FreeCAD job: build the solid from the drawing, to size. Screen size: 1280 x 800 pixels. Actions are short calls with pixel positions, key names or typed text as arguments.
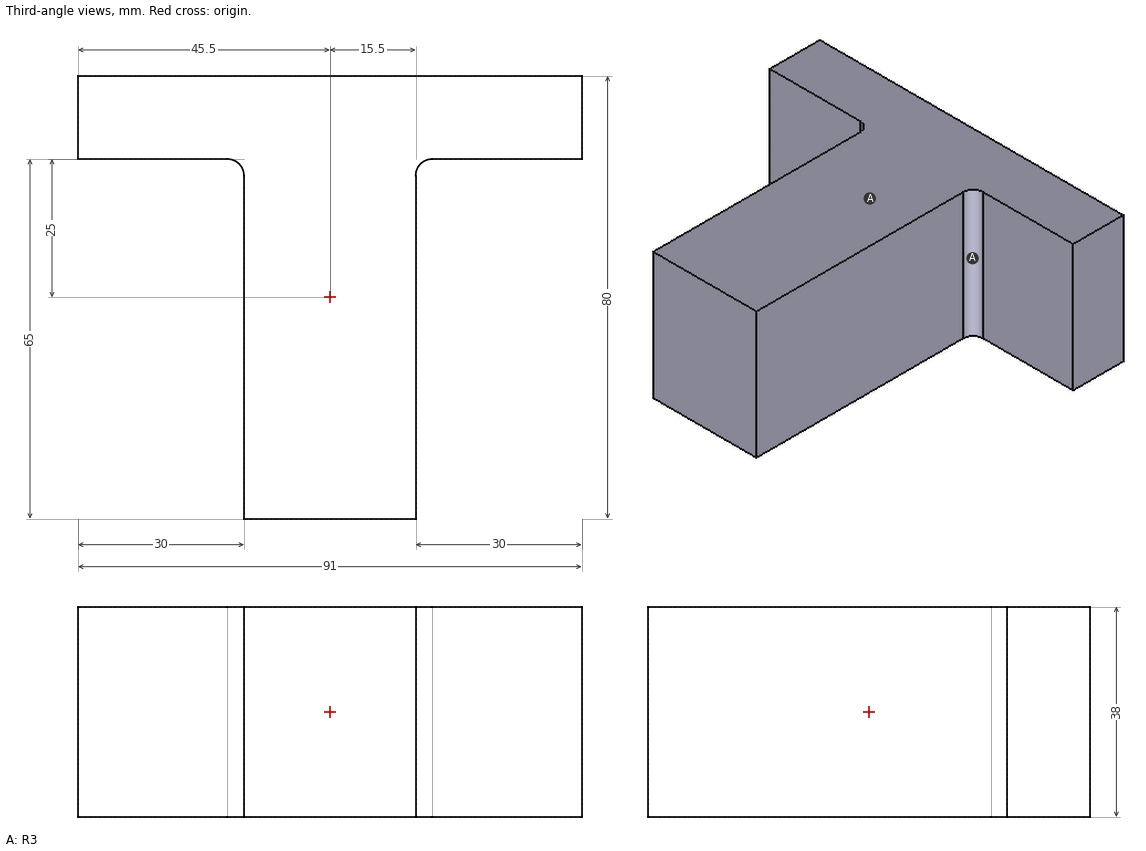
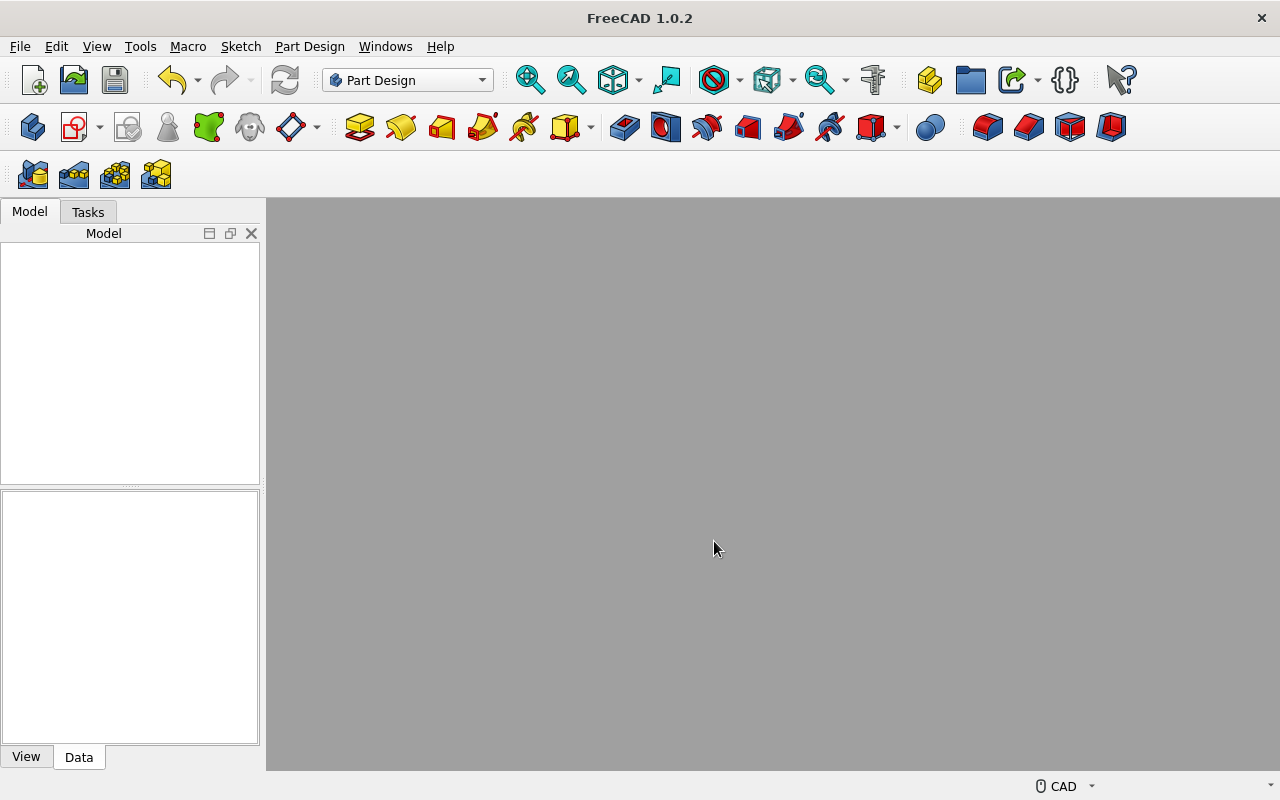
click(33, 80)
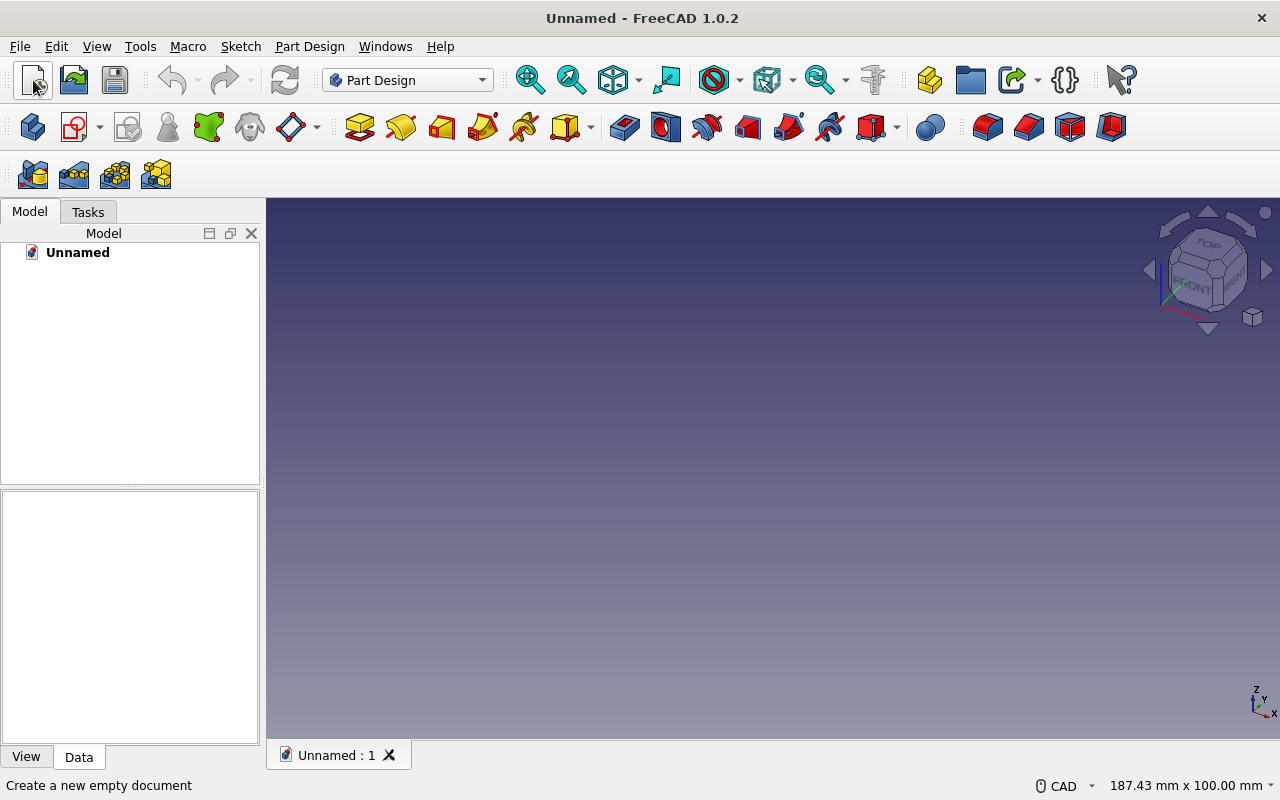
click(74, 128)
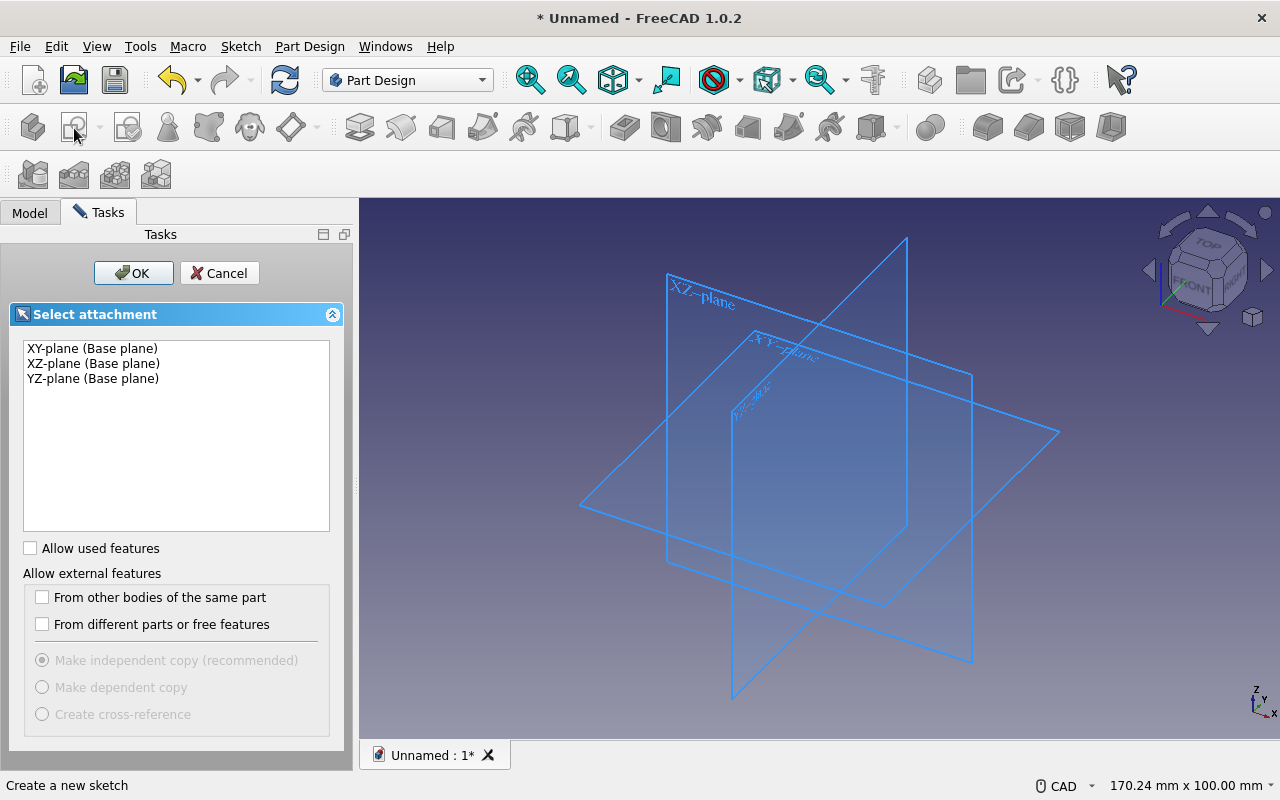
click(84, 348)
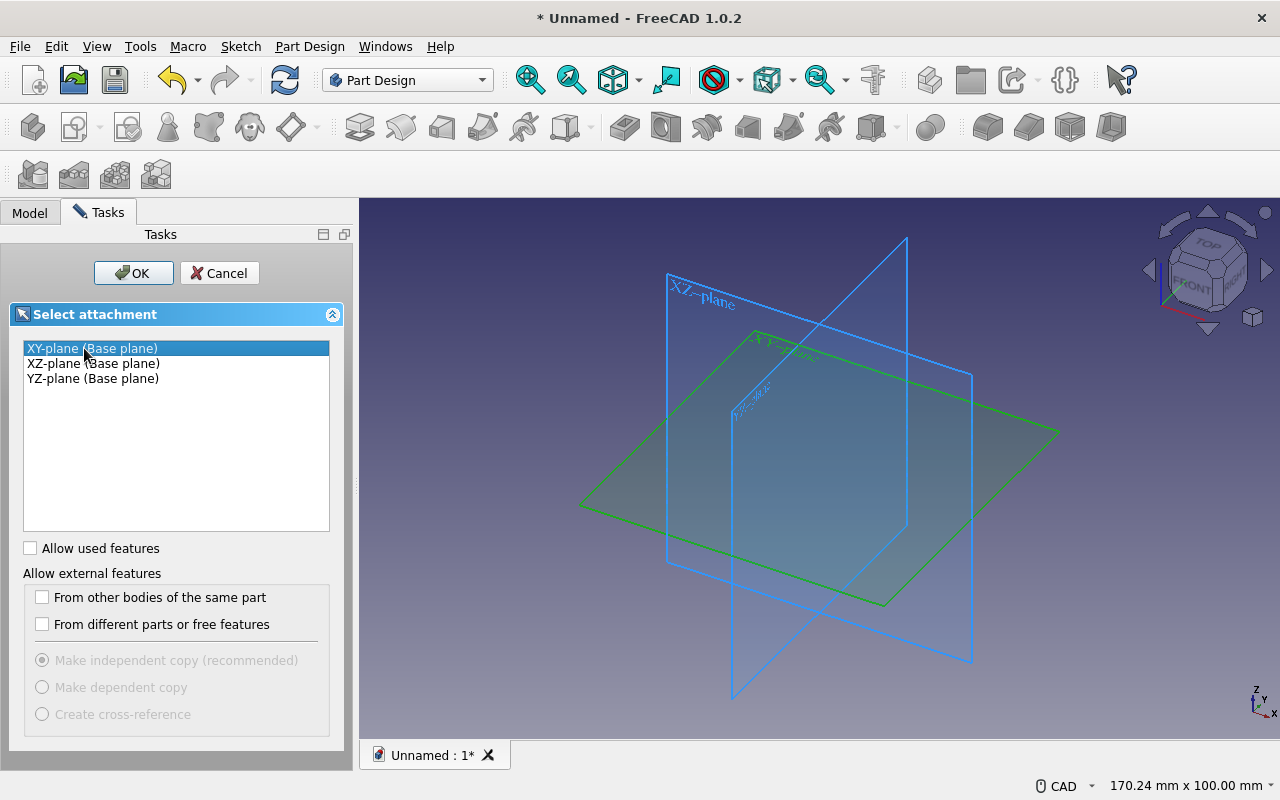
click(134, 273)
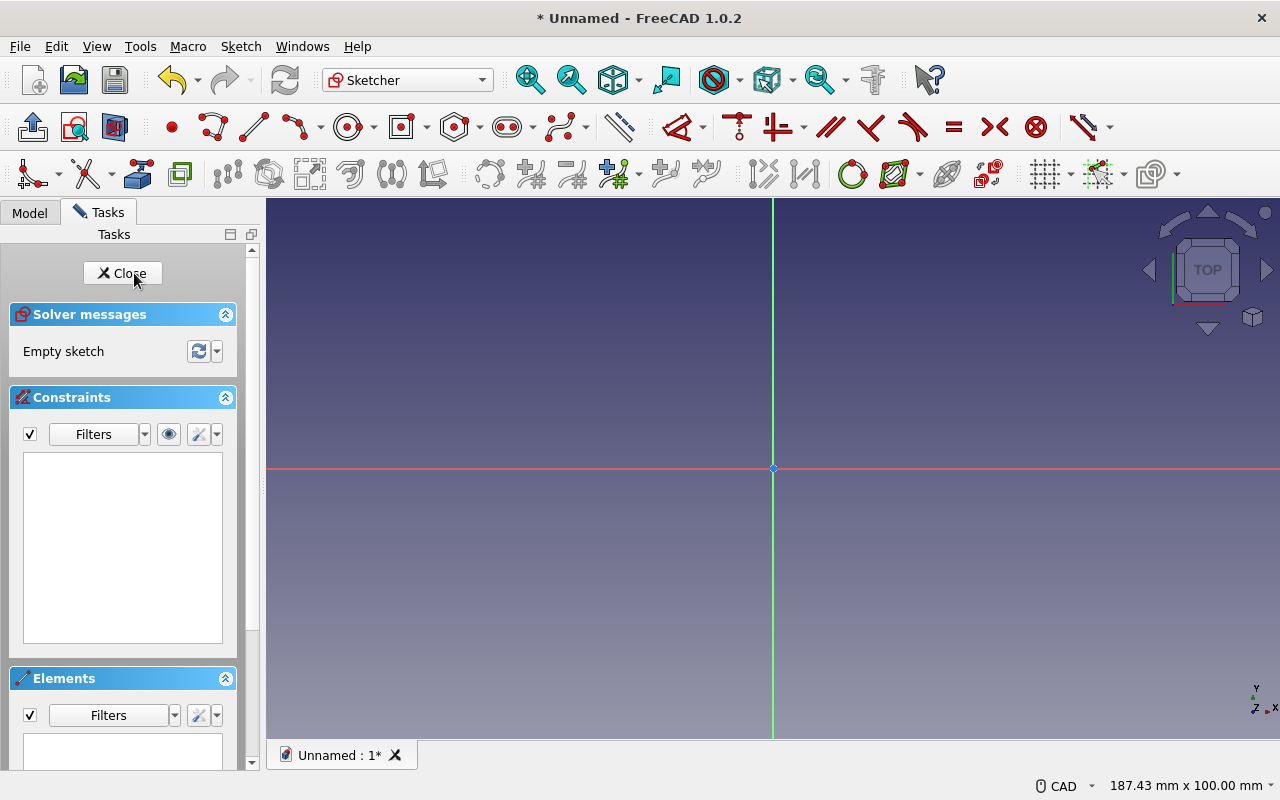
click(400, 128)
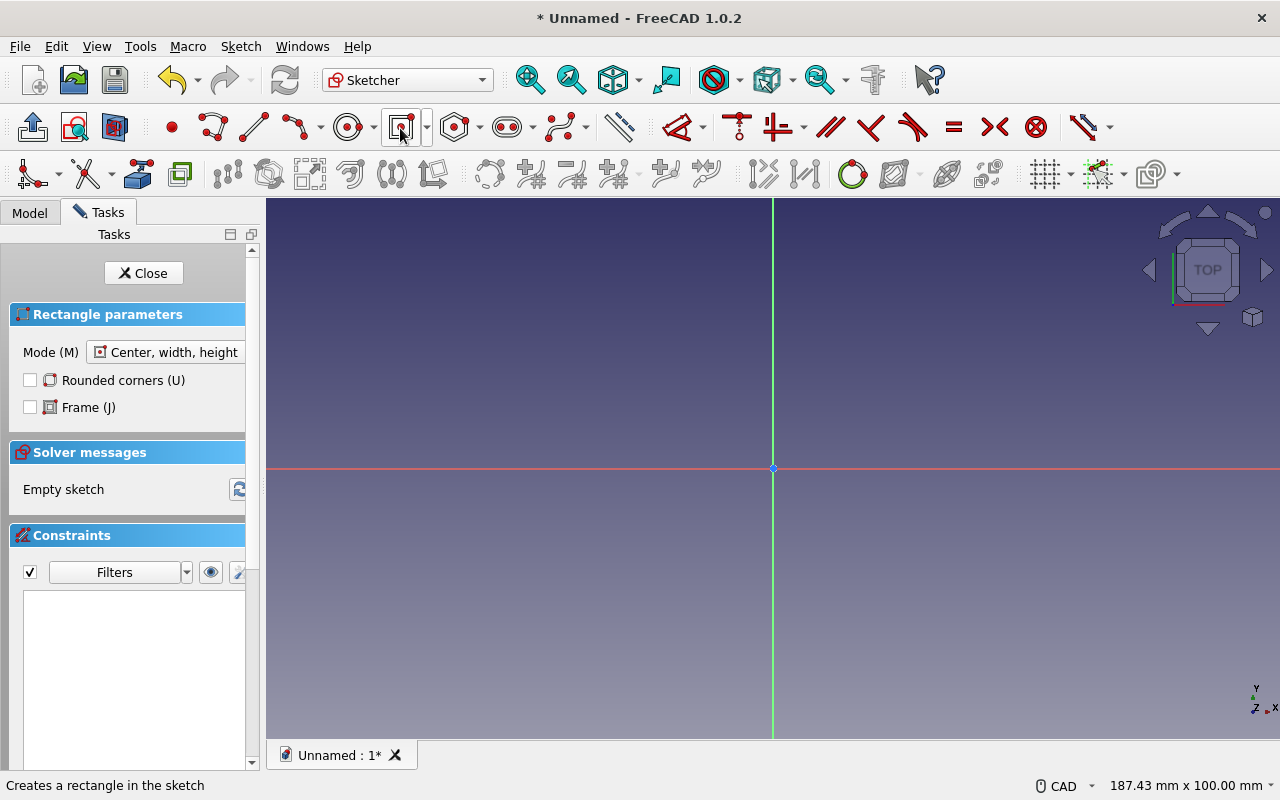
click(773, 468)
move(1019, 252)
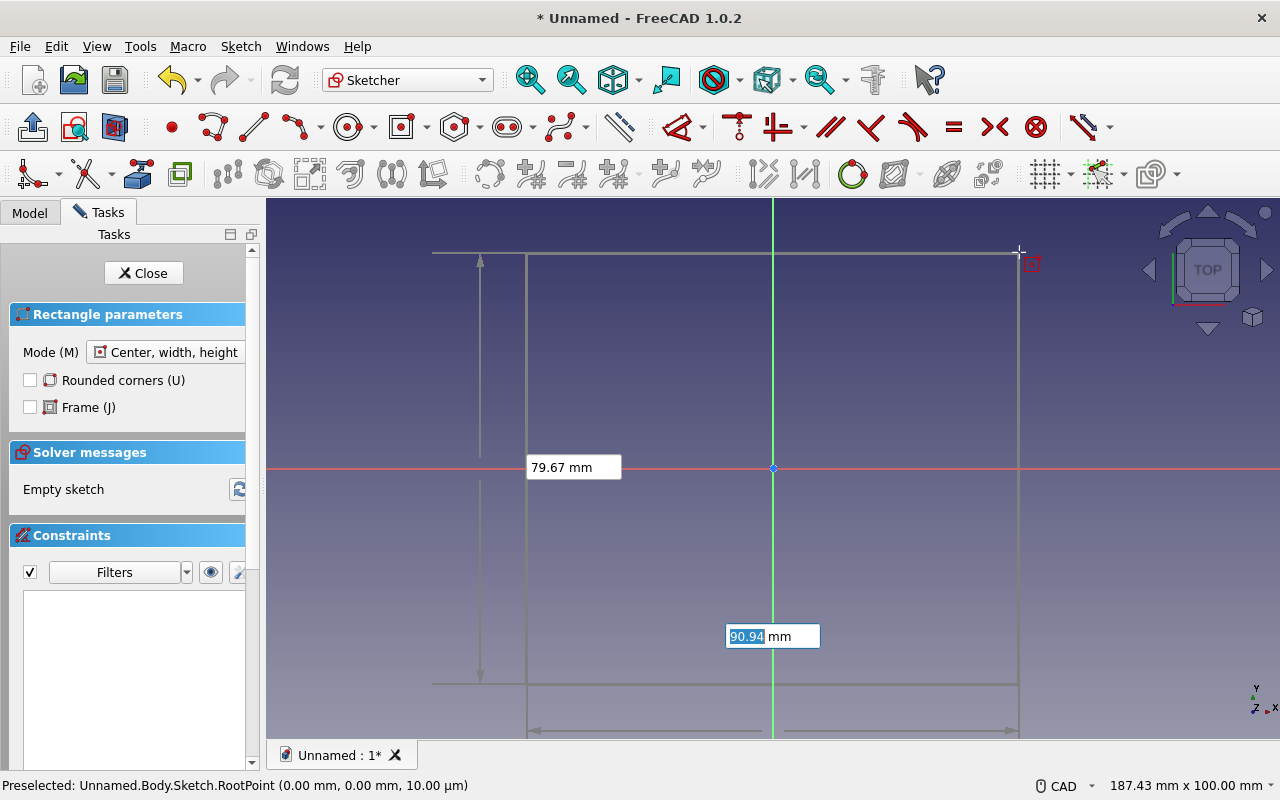
text(91)
key(Tab)
text(80)
key(Return)
key(Escape)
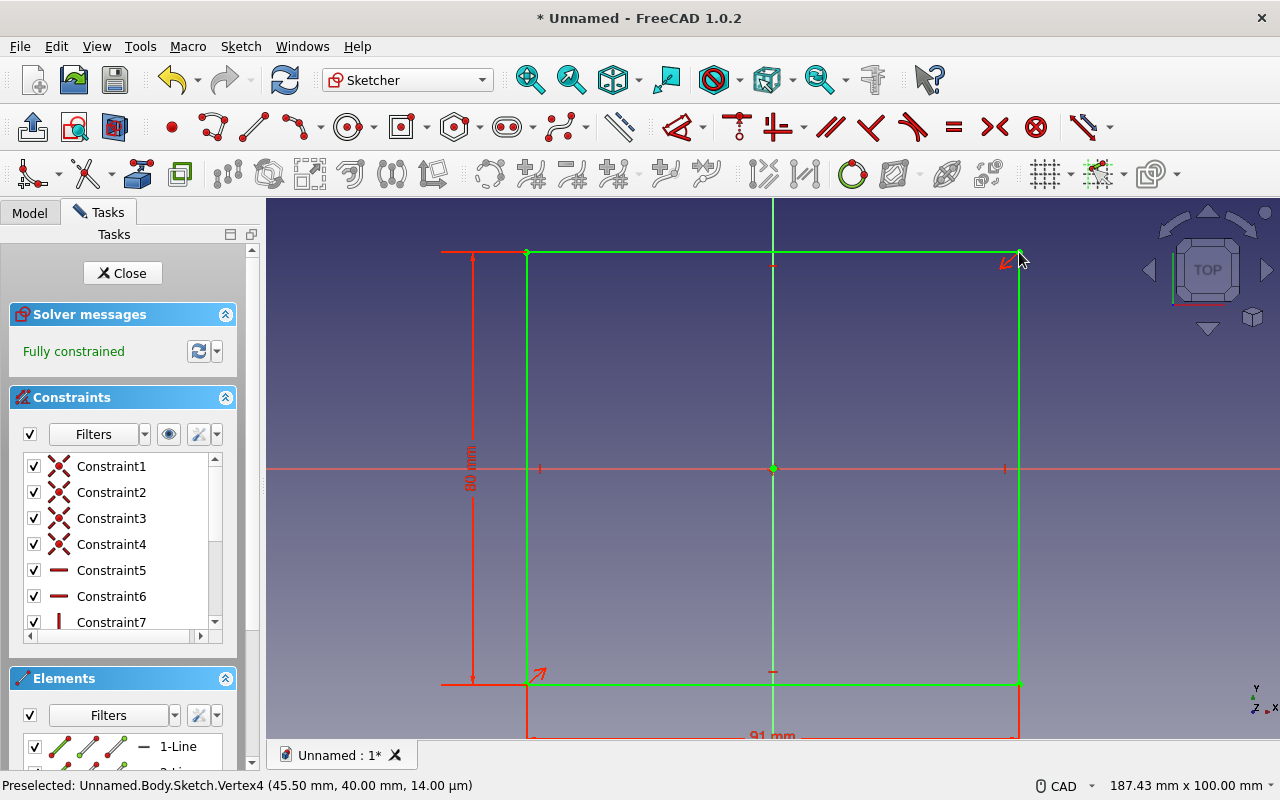
click(123, 273)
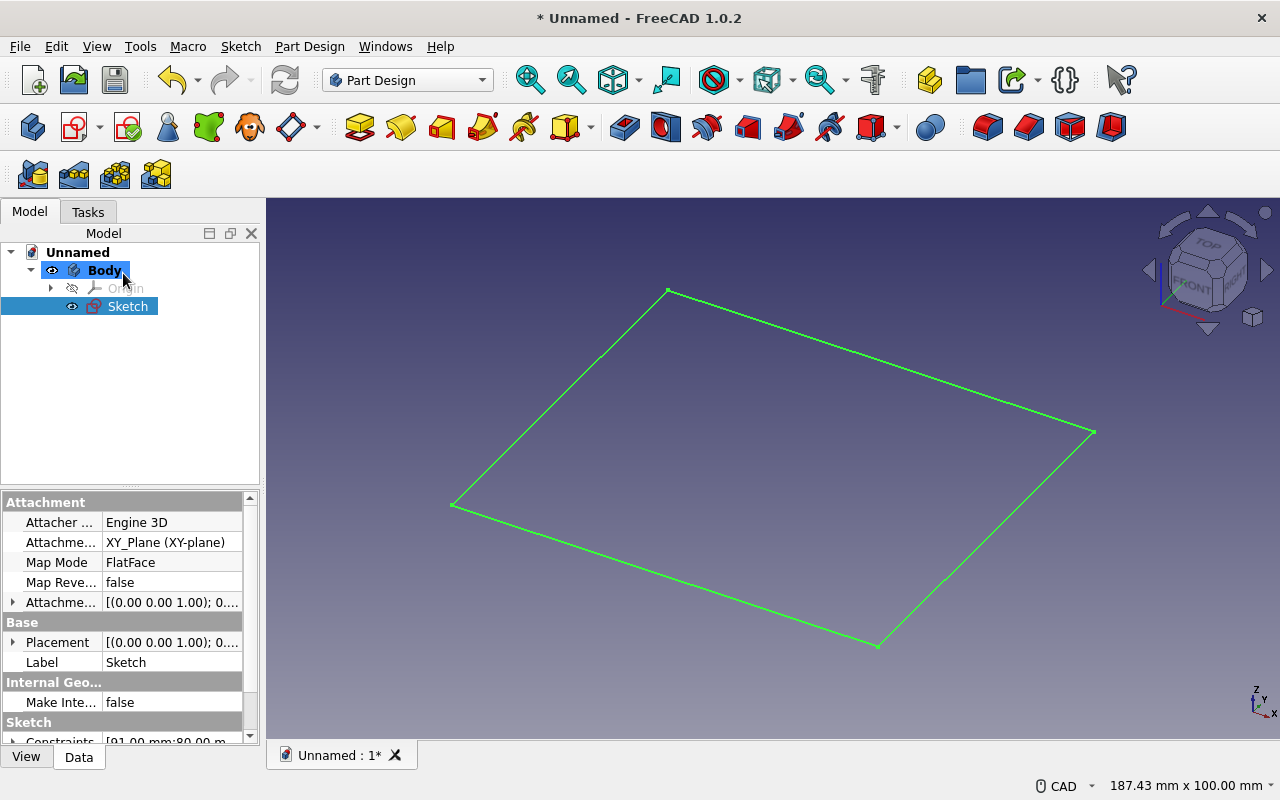
click(360, 128)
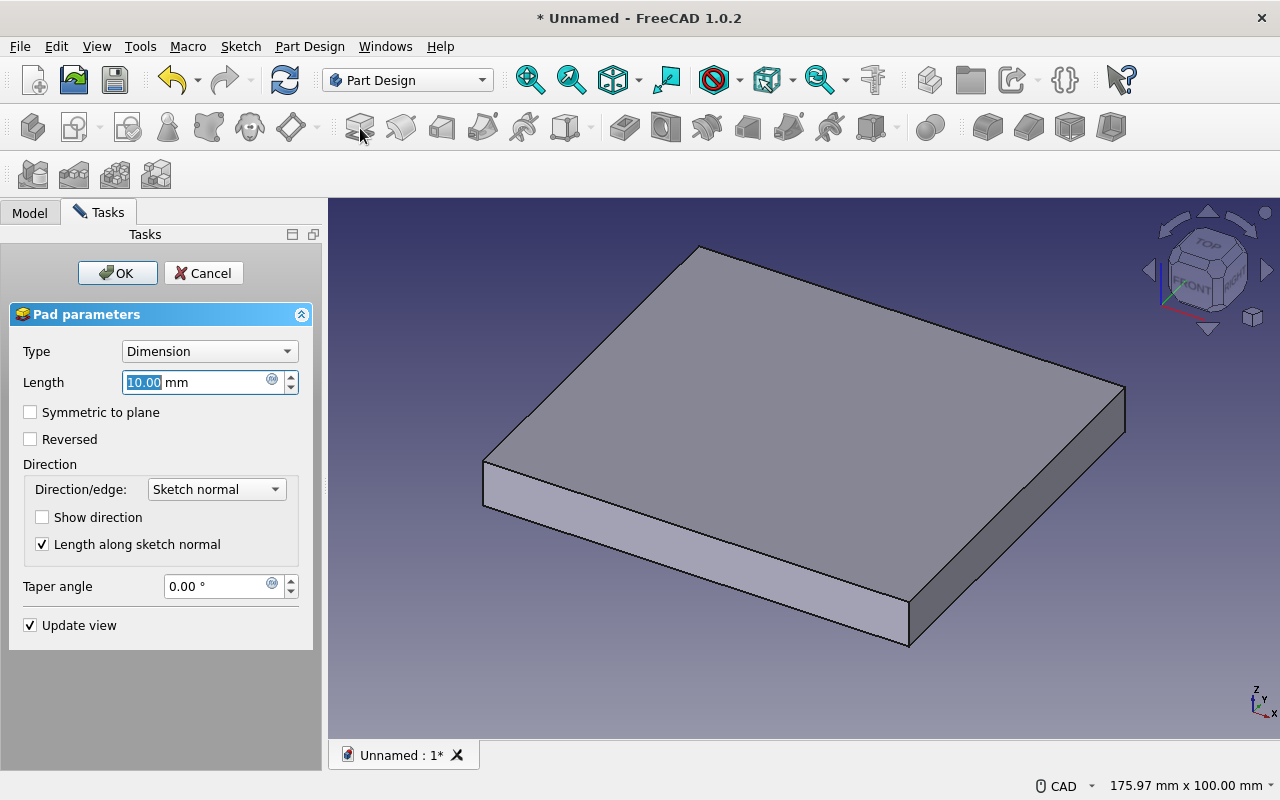
text(38)
key(Tab)